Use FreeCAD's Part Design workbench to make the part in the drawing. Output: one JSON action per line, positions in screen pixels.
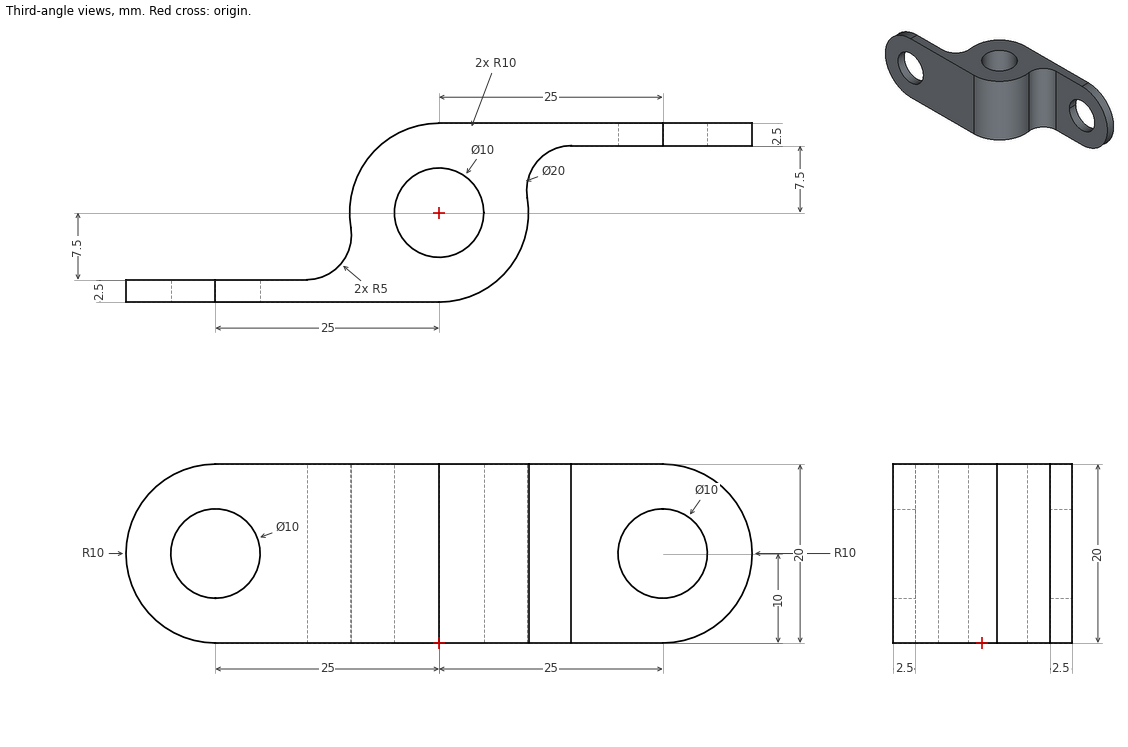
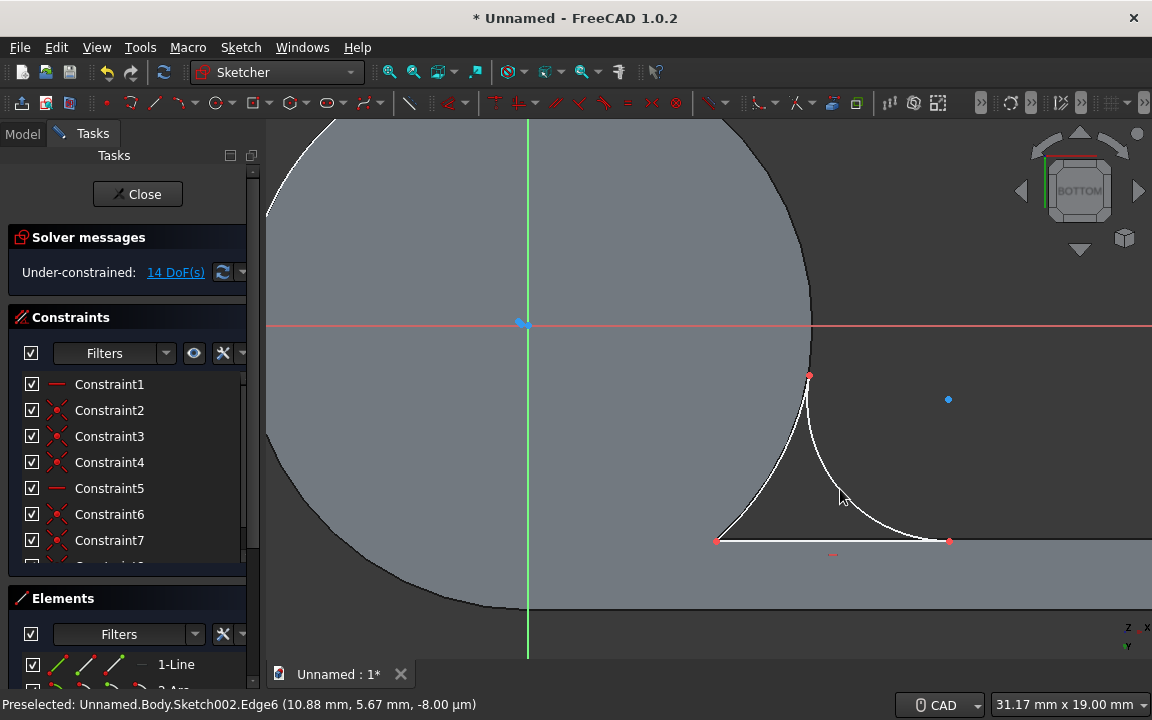
{"action": "scroll", "coordinate": [777, 466], "scroll_direction": "down", "scroll_amount": 3}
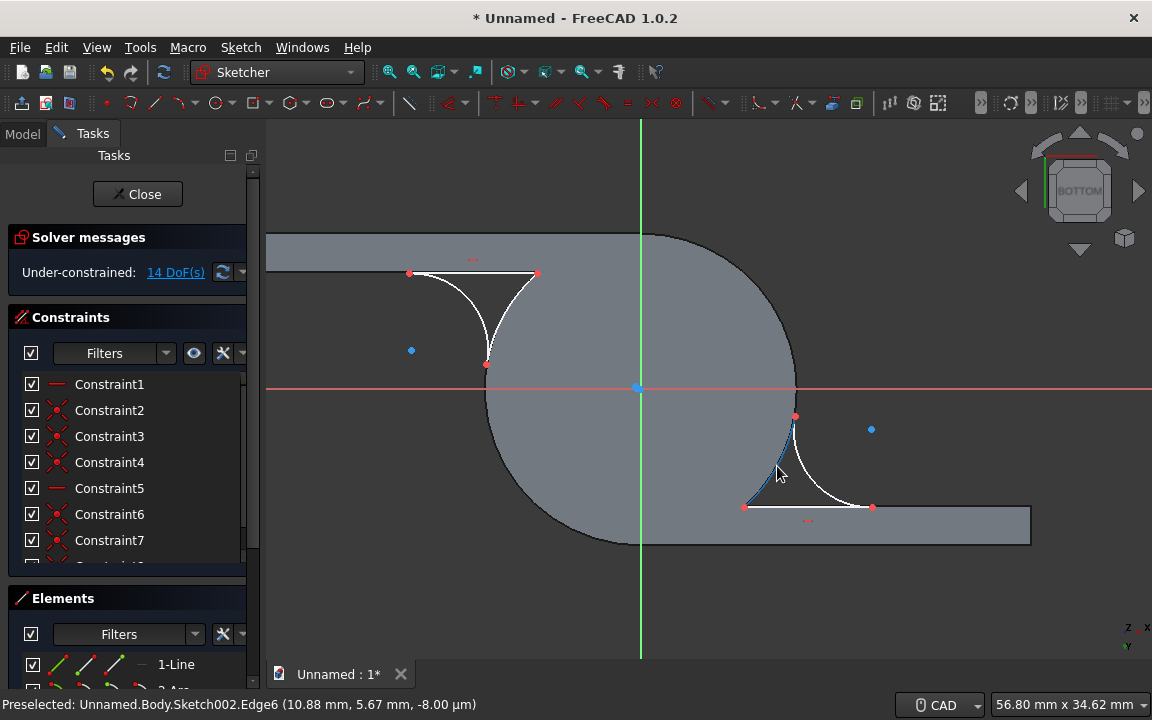
{"action": "scroll", "coordinate": [448, 273], "scroll_direction": "up", "scroll_amount": 3}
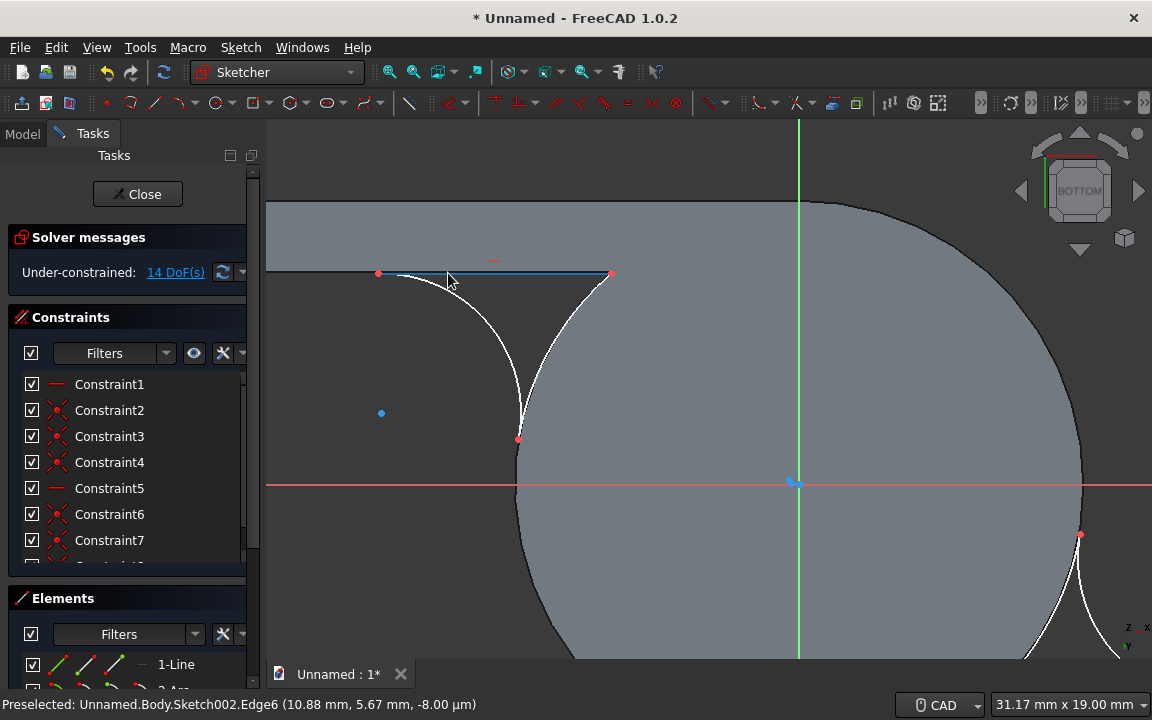
{"action": "left_click", "coordinate": [448, 274]}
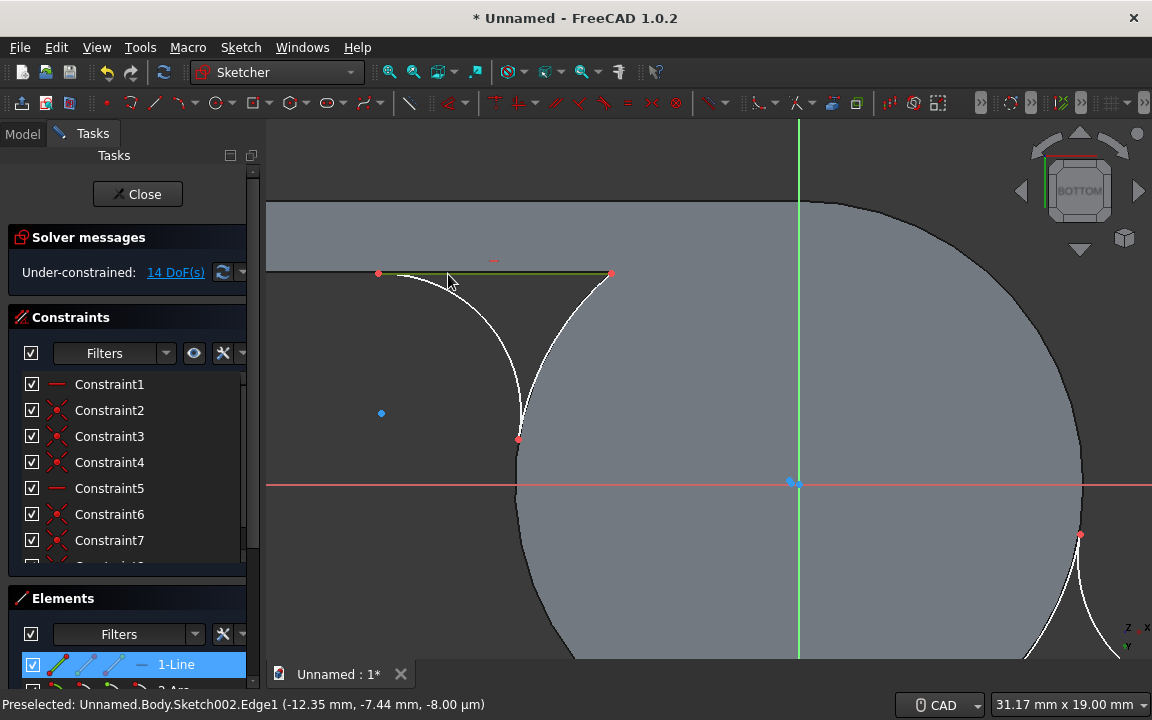
{"action": "left_click", "coordinate": [513, 366]}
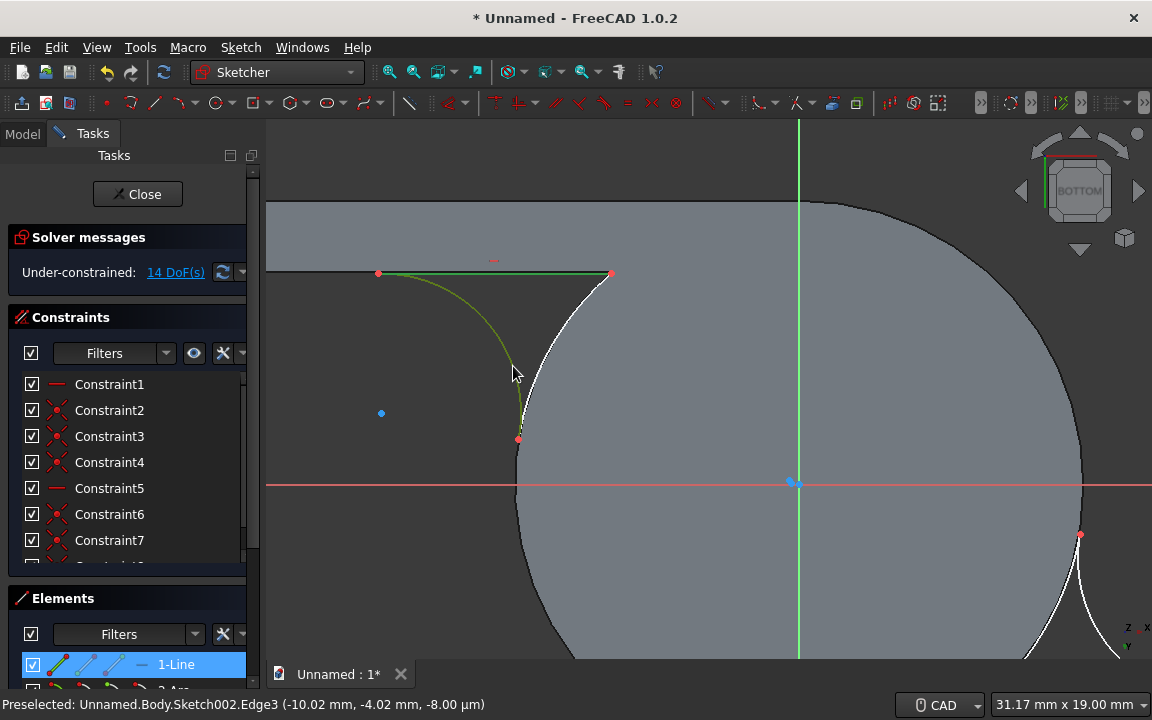
{"action": "key", "text": "t"}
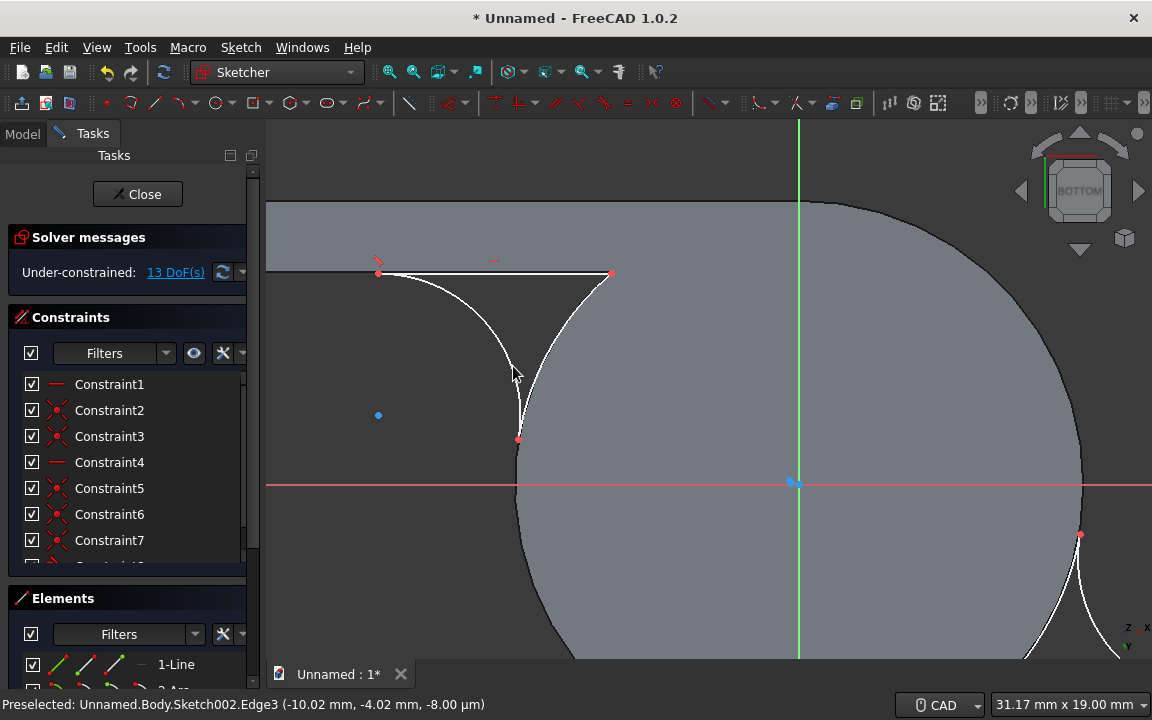
{"action": "left_click", "coordinate": [572, 316]}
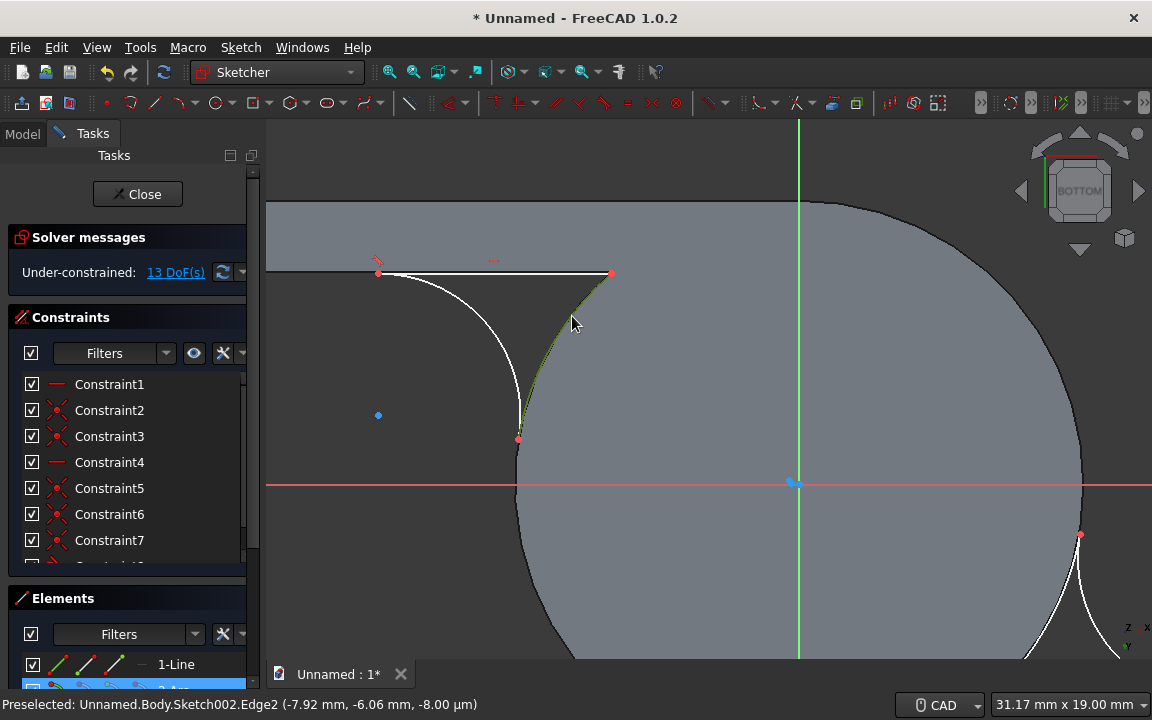
{"action": "left_click", "coordinate": [512, 366]}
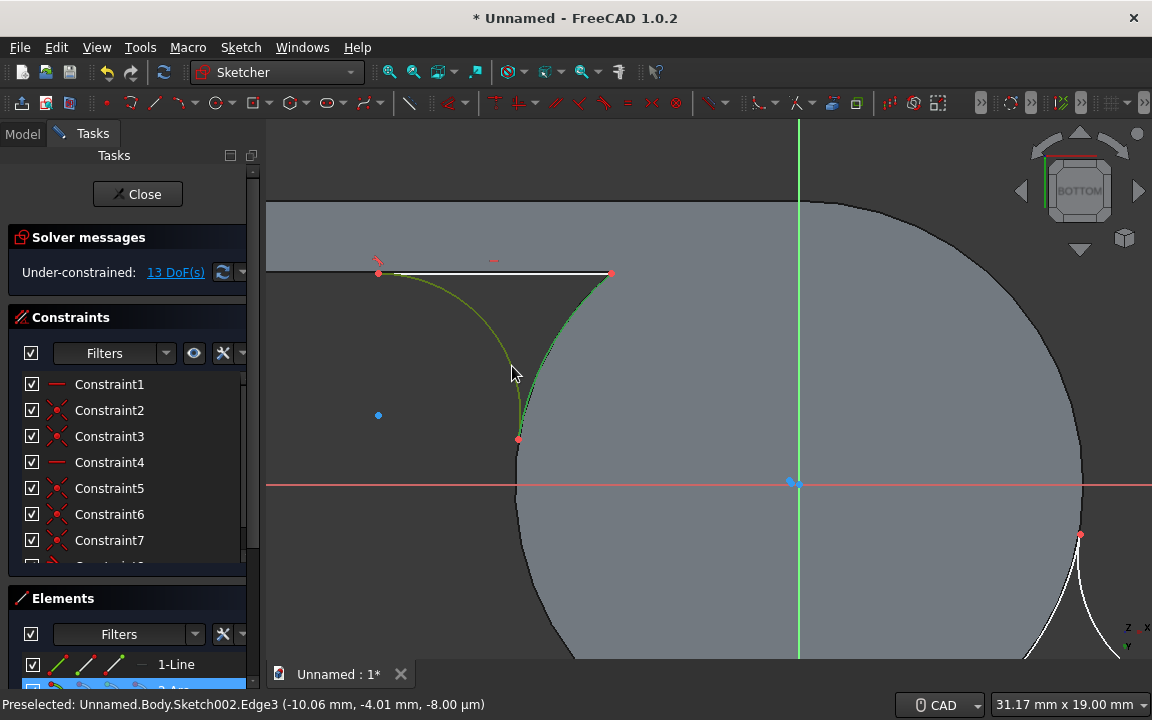
{"action": "key", "text": "t"}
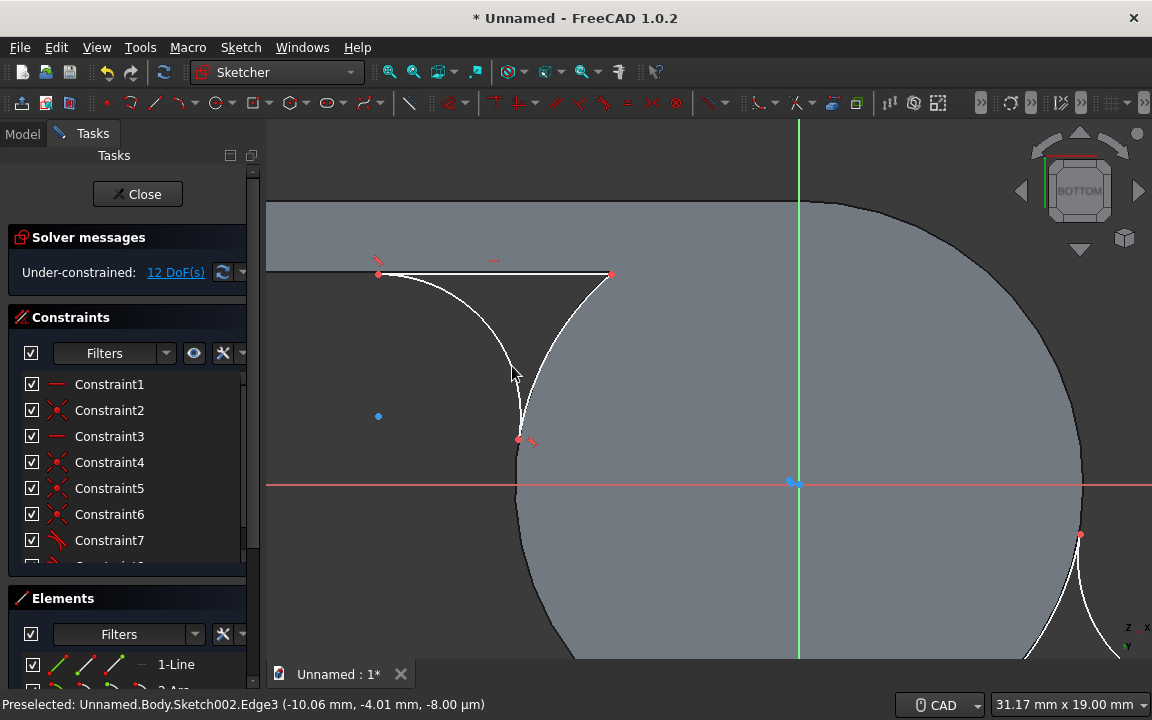
{"action": "scroll", "coordinate": [448, 272], "scroll_direction": "down", "scroll_amount": 3}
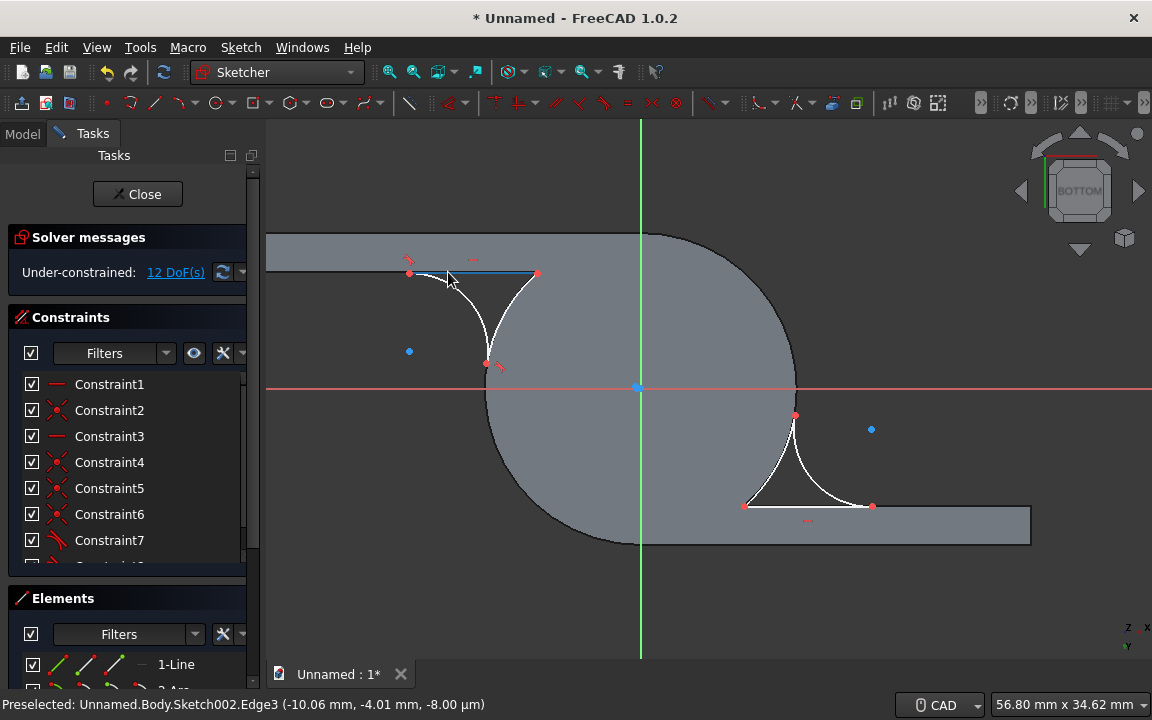
{"action": "scroll", "coordinate": [834, 507], "scroll_direction": "up", "scroll_amount": 3}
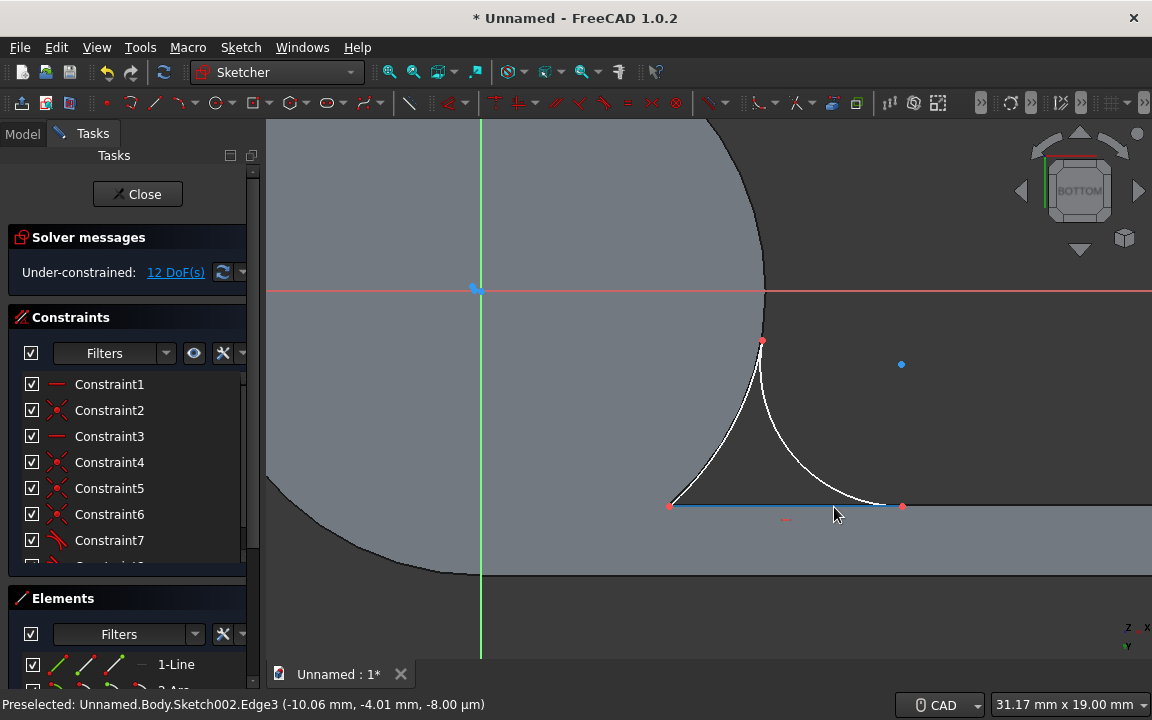
{"action": "left_click", "coordinate": [833, 506]}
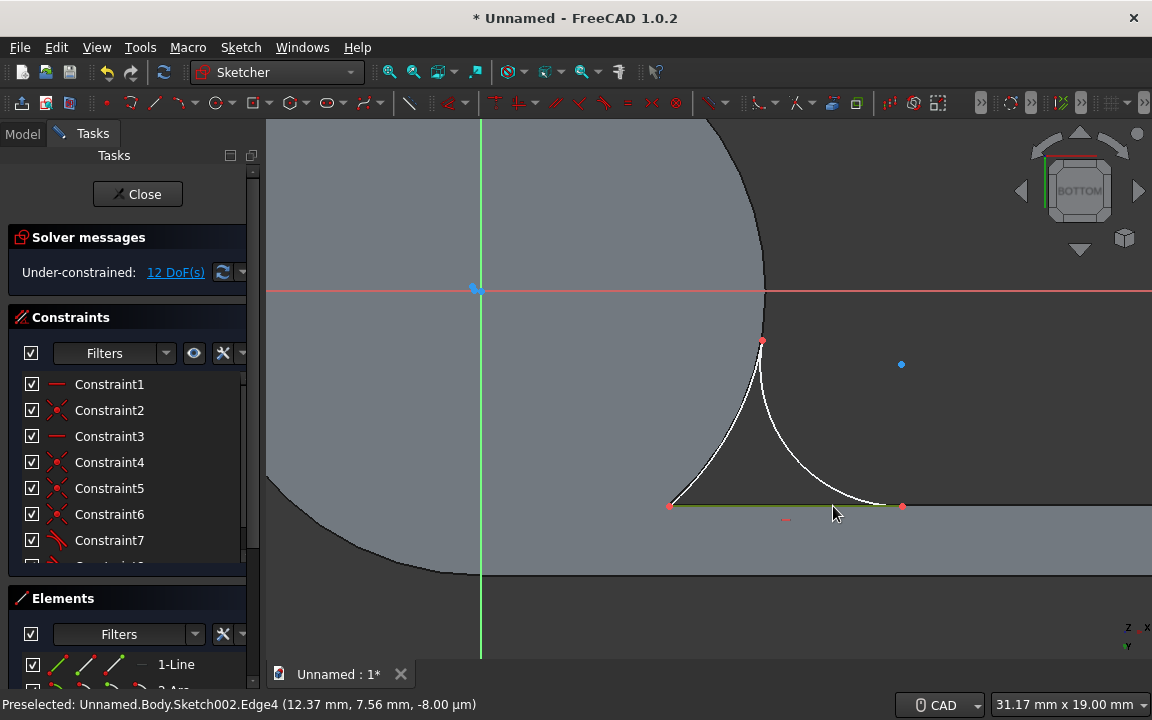
{"action": "left_click", "coordinate": [769, 414]}